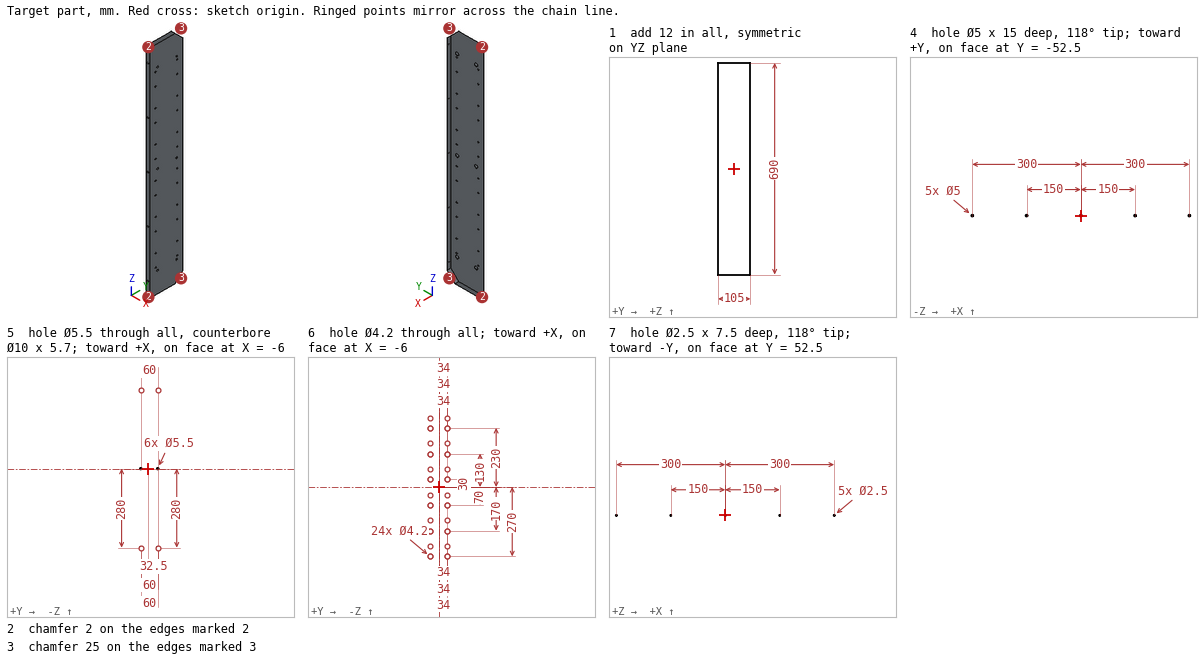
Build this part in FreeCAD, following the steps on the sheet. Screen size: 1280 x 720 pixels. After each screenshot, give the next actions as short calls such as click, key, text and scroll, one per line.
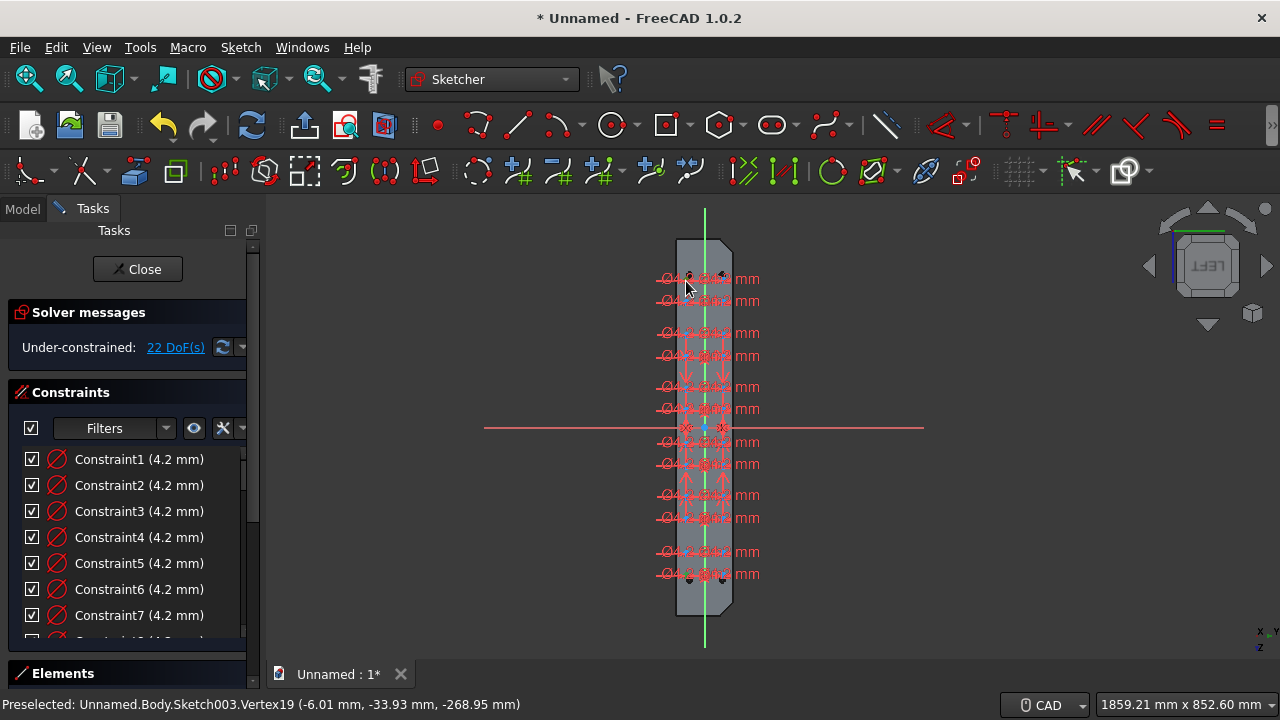
click(529, 428)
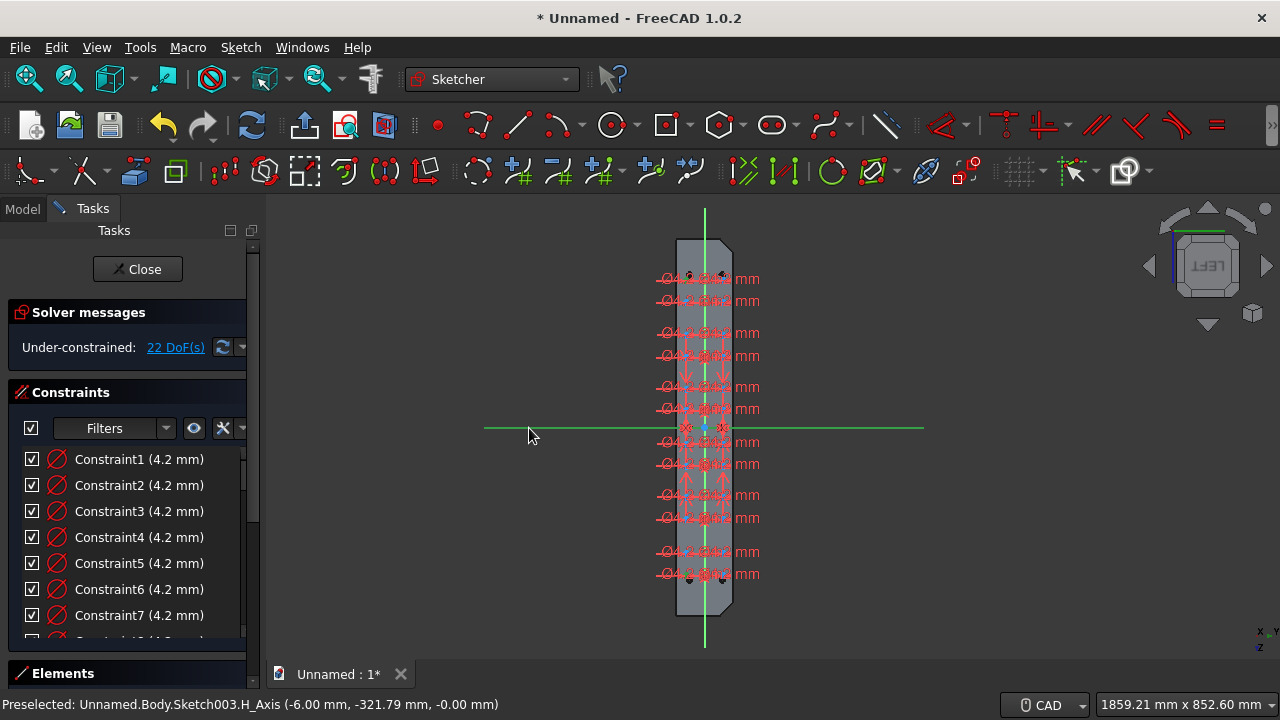
key(s)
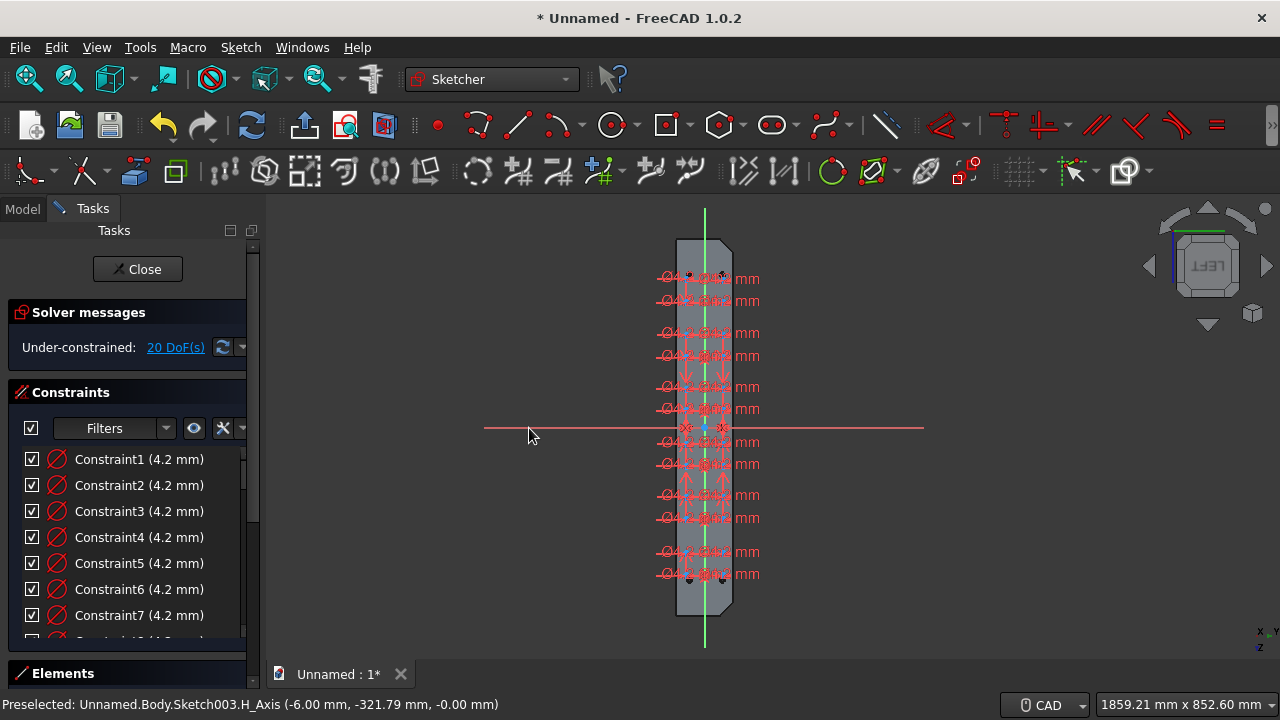
click(723, 576)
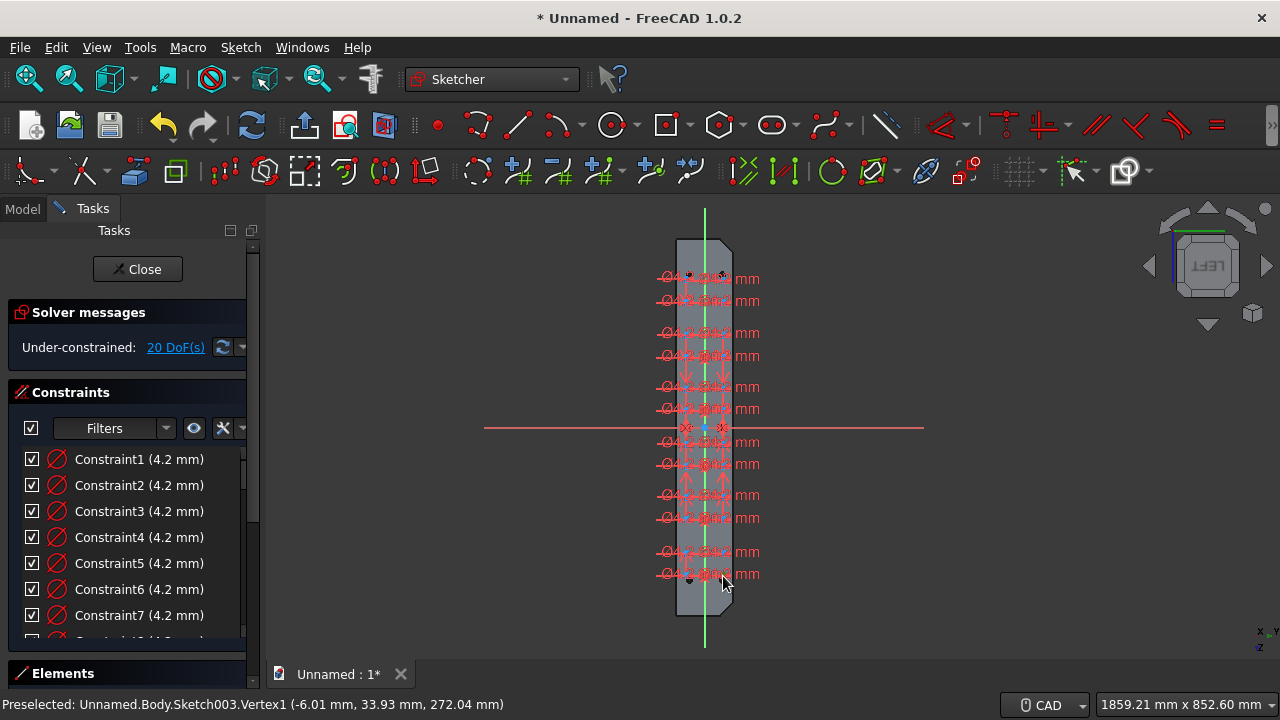
click(723, 281)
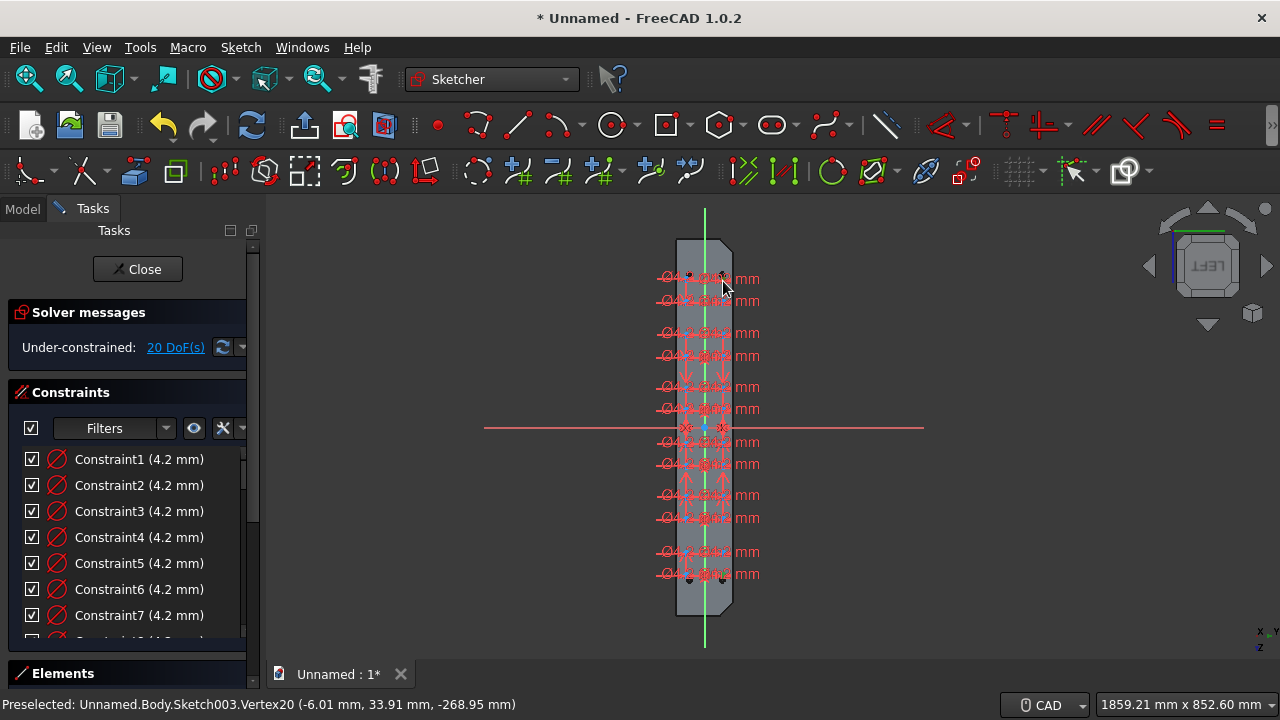
click(529, 428)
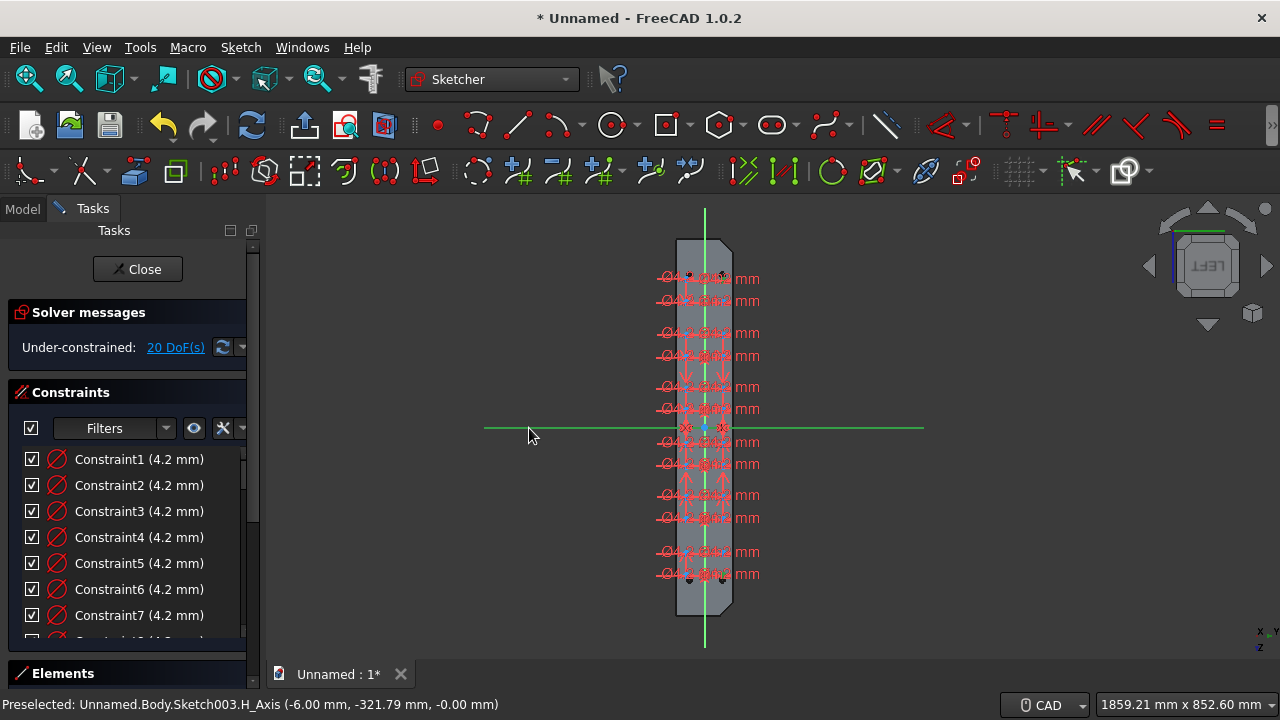
key(s)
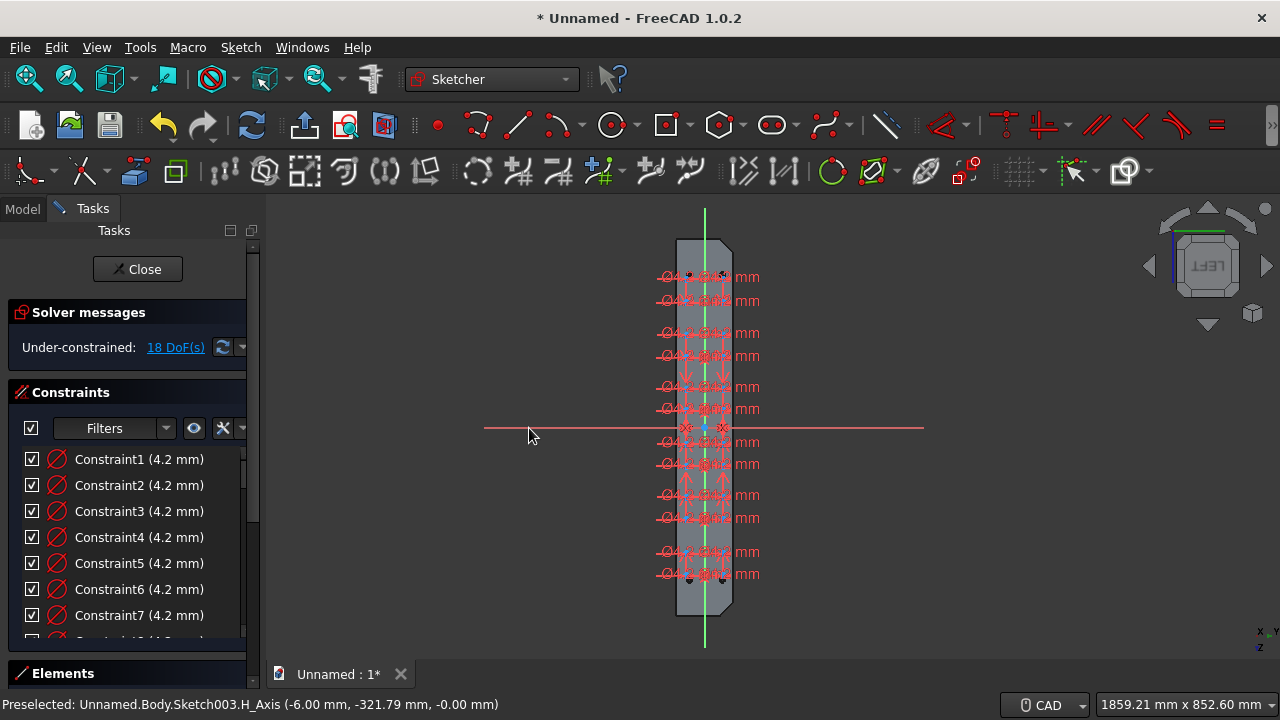
click(723, 303)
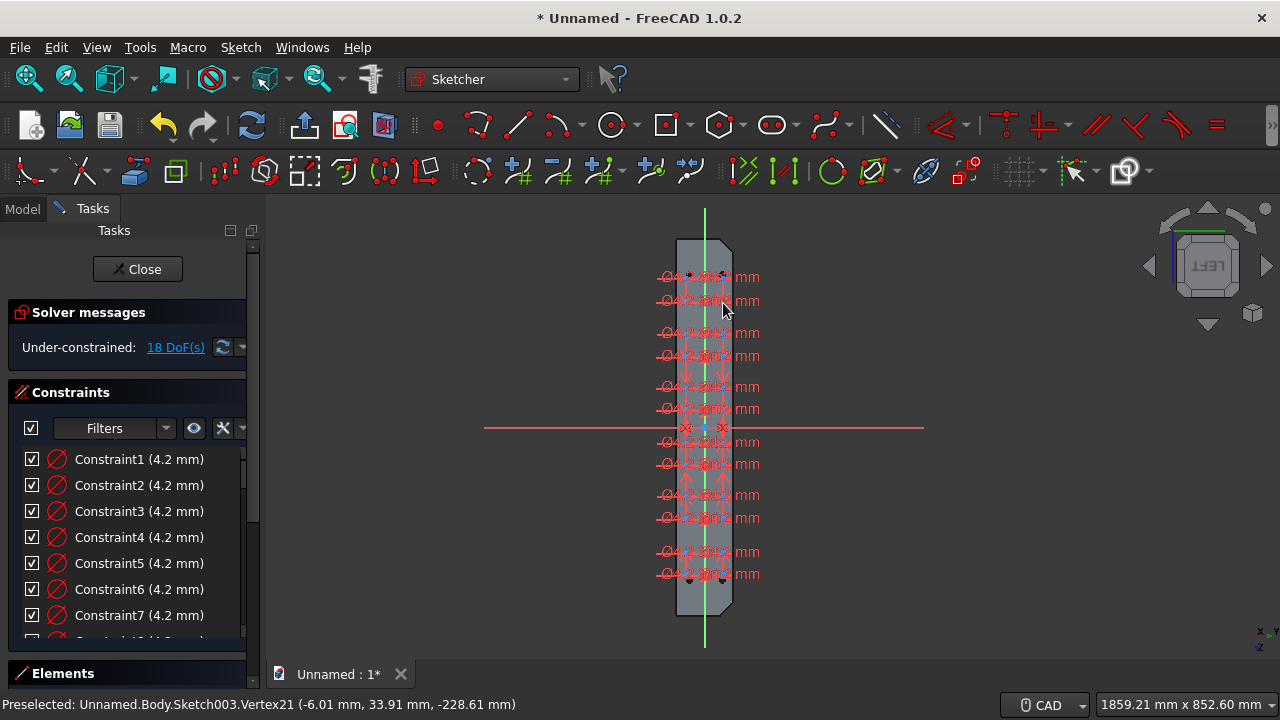
click(686, 303)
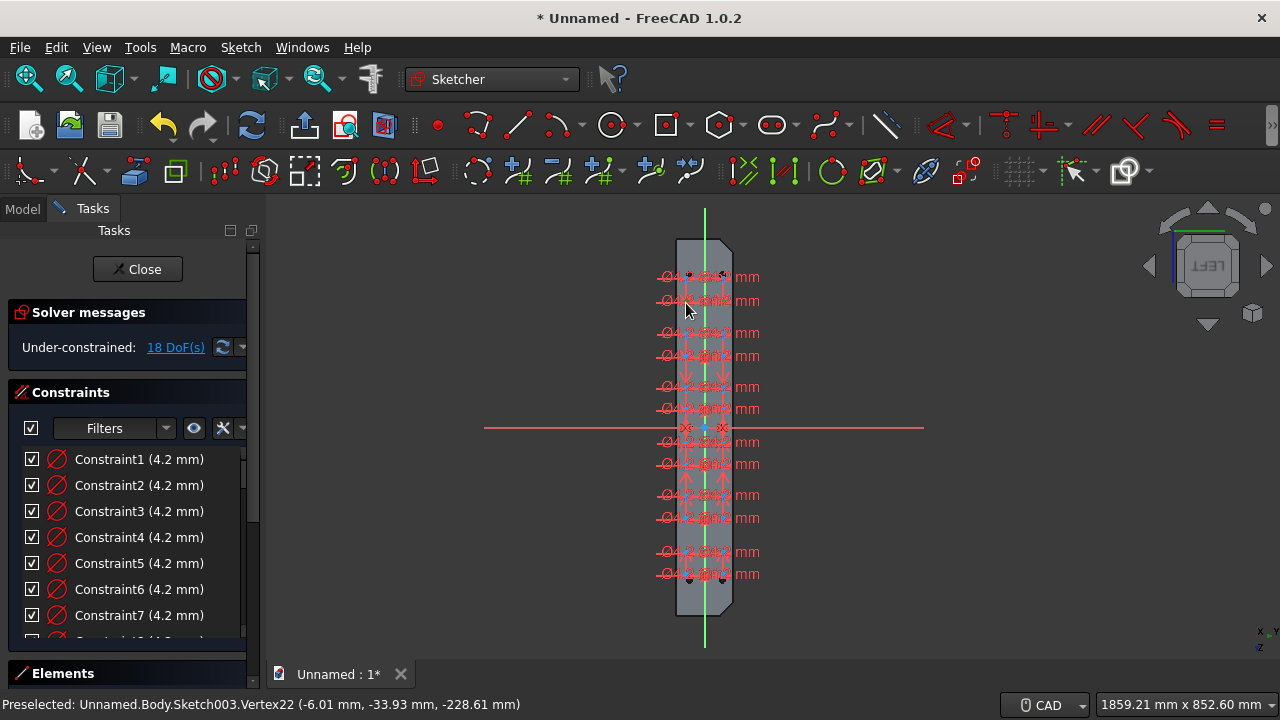
click(705, 602)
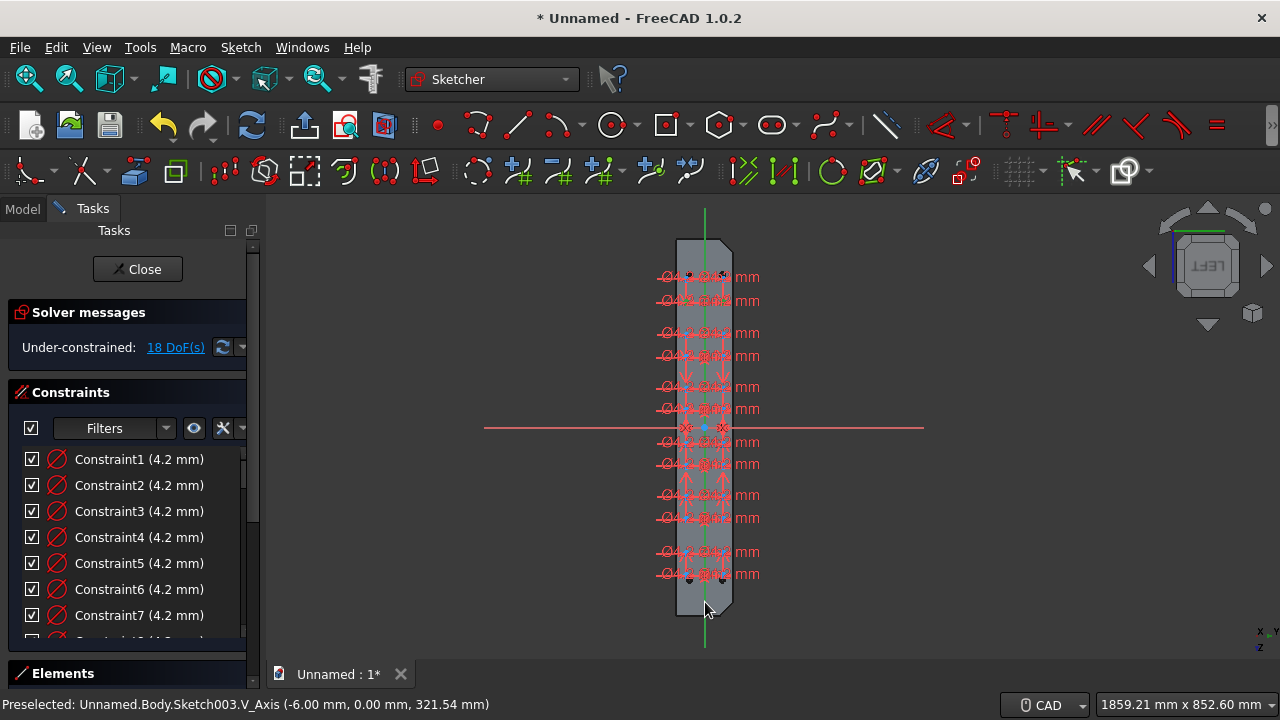
key(s)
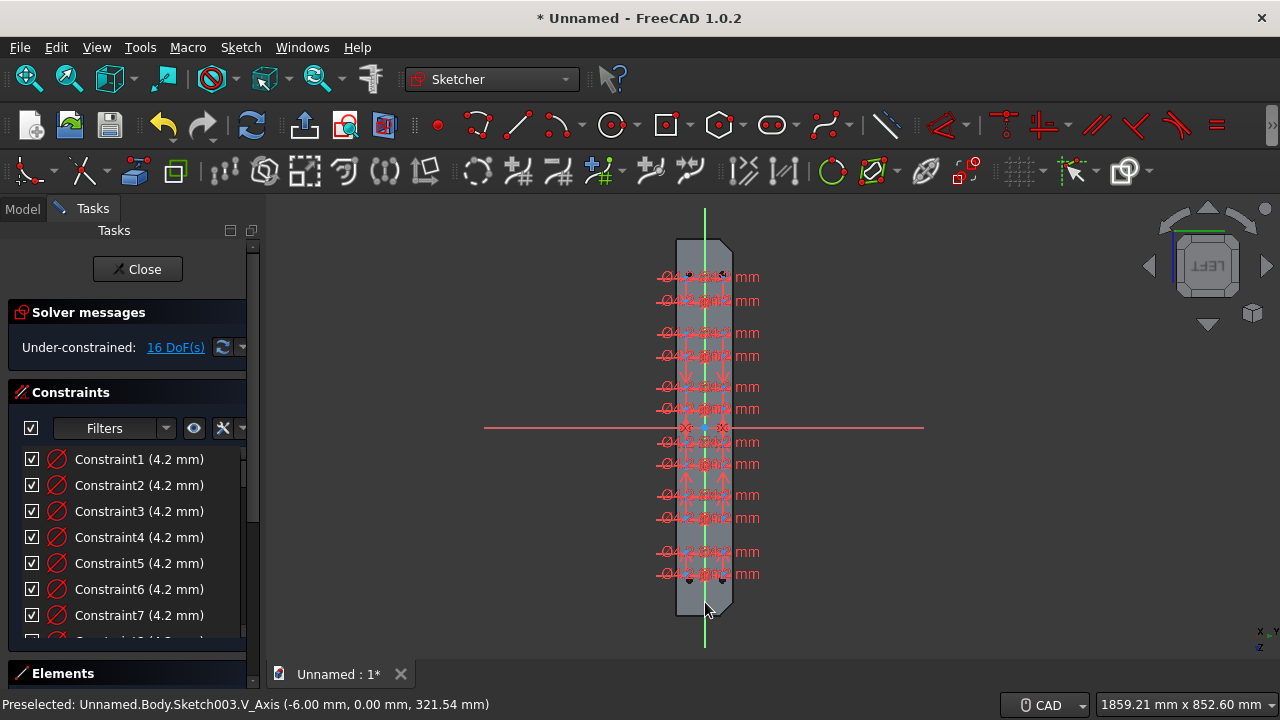
click(686, 303)